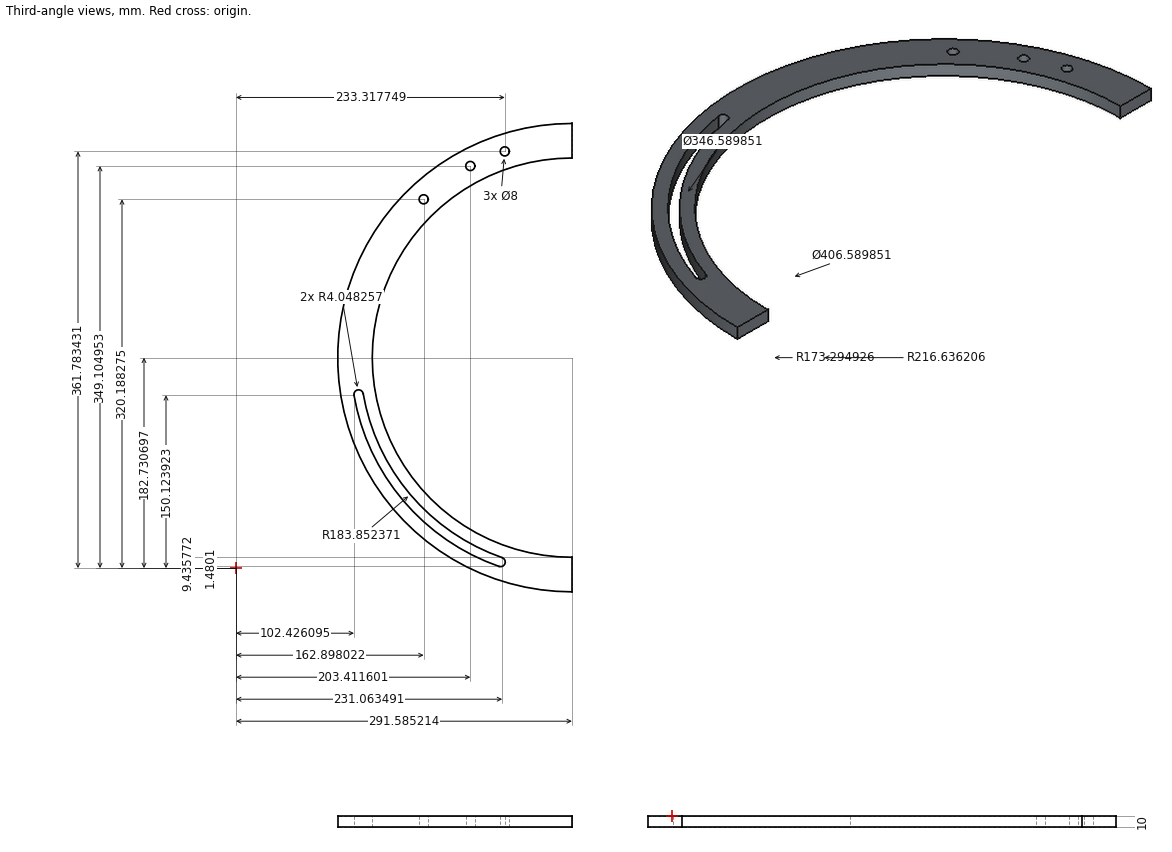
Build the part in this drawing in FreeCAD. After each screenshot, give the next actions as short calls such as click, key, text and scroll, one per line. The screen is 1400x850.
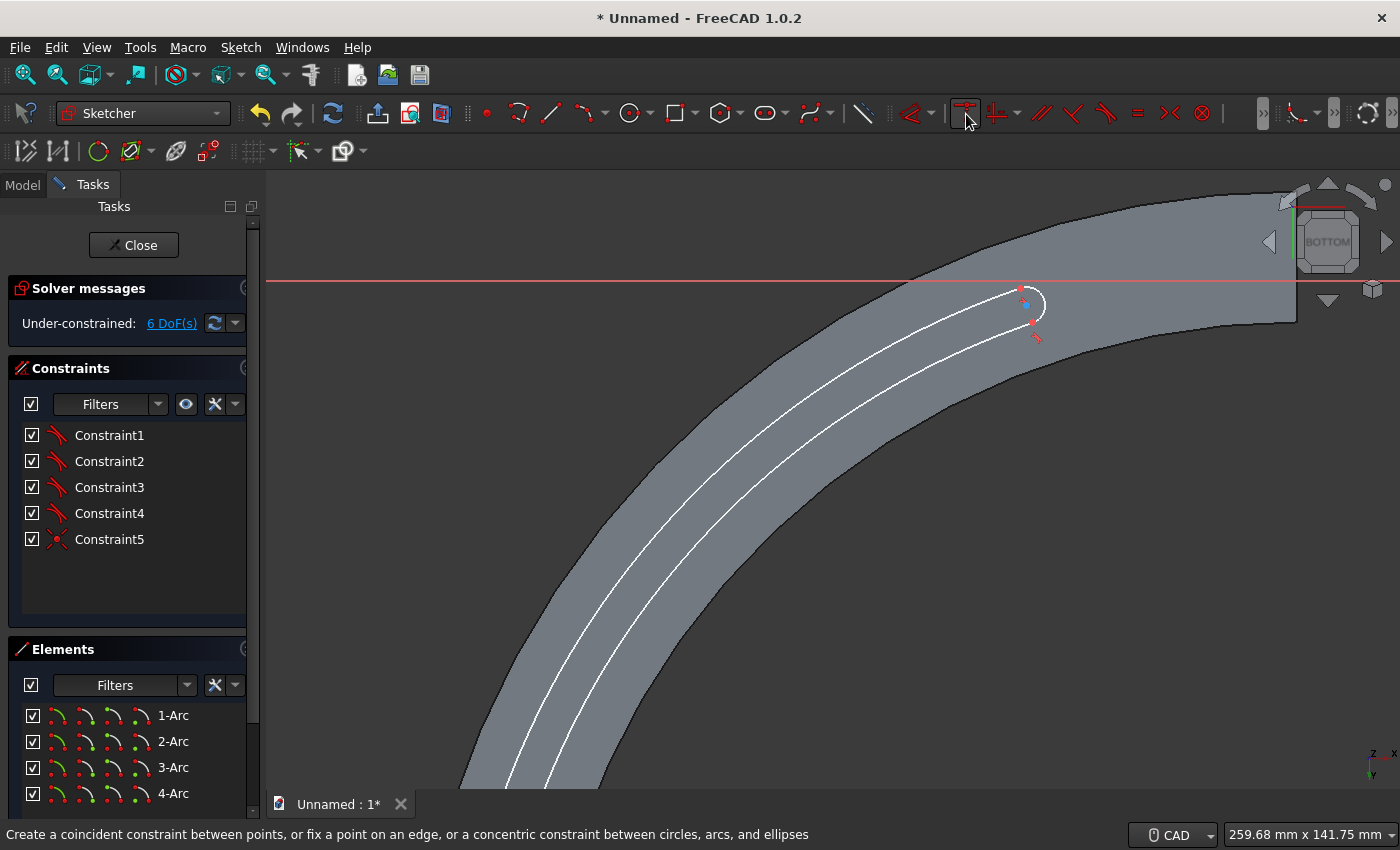
click(910, 114)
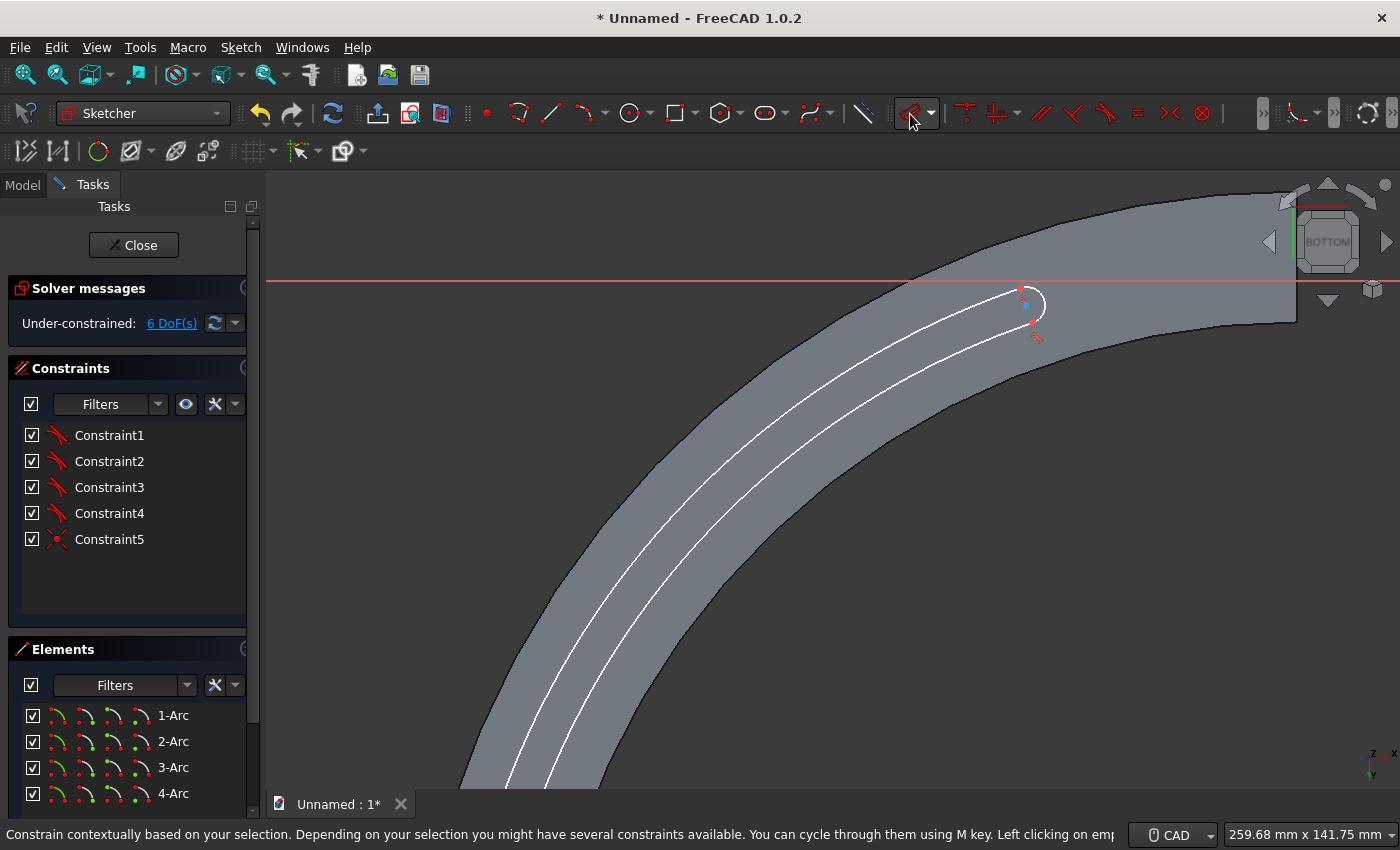
scroll(1046, 310, down, 3)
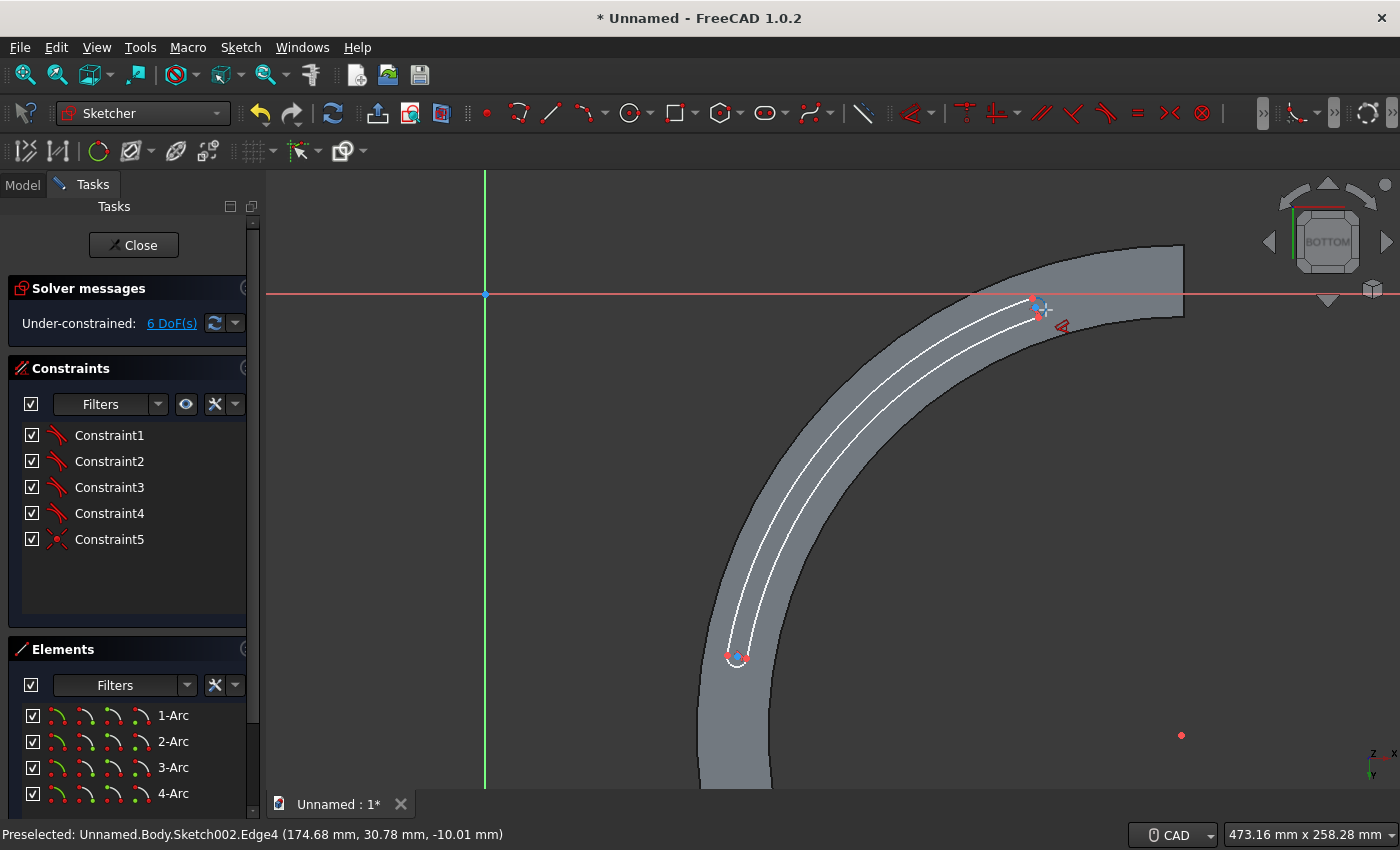
scroll(730, 664, up, 8)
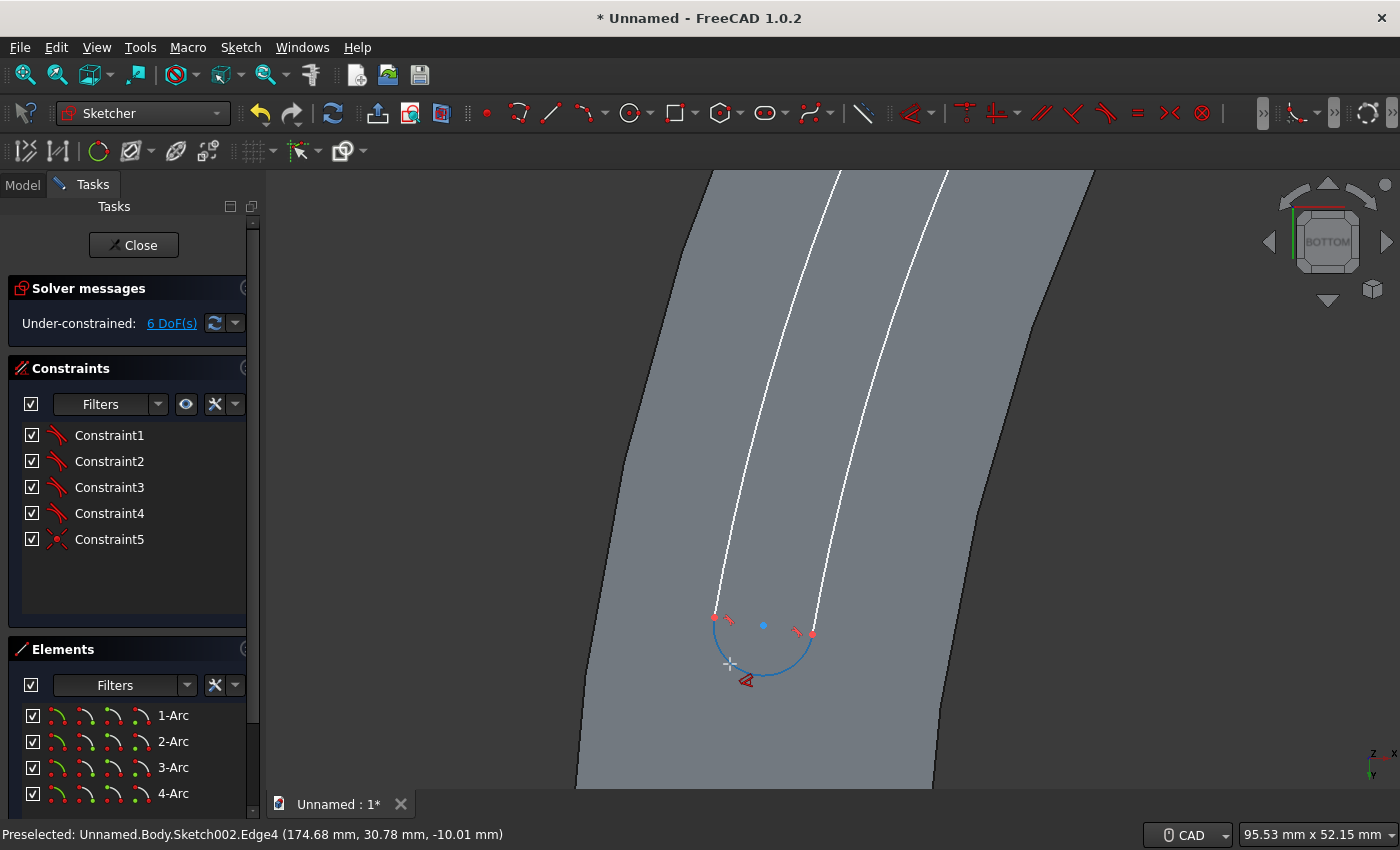
click(728, 660)
click(705, 682)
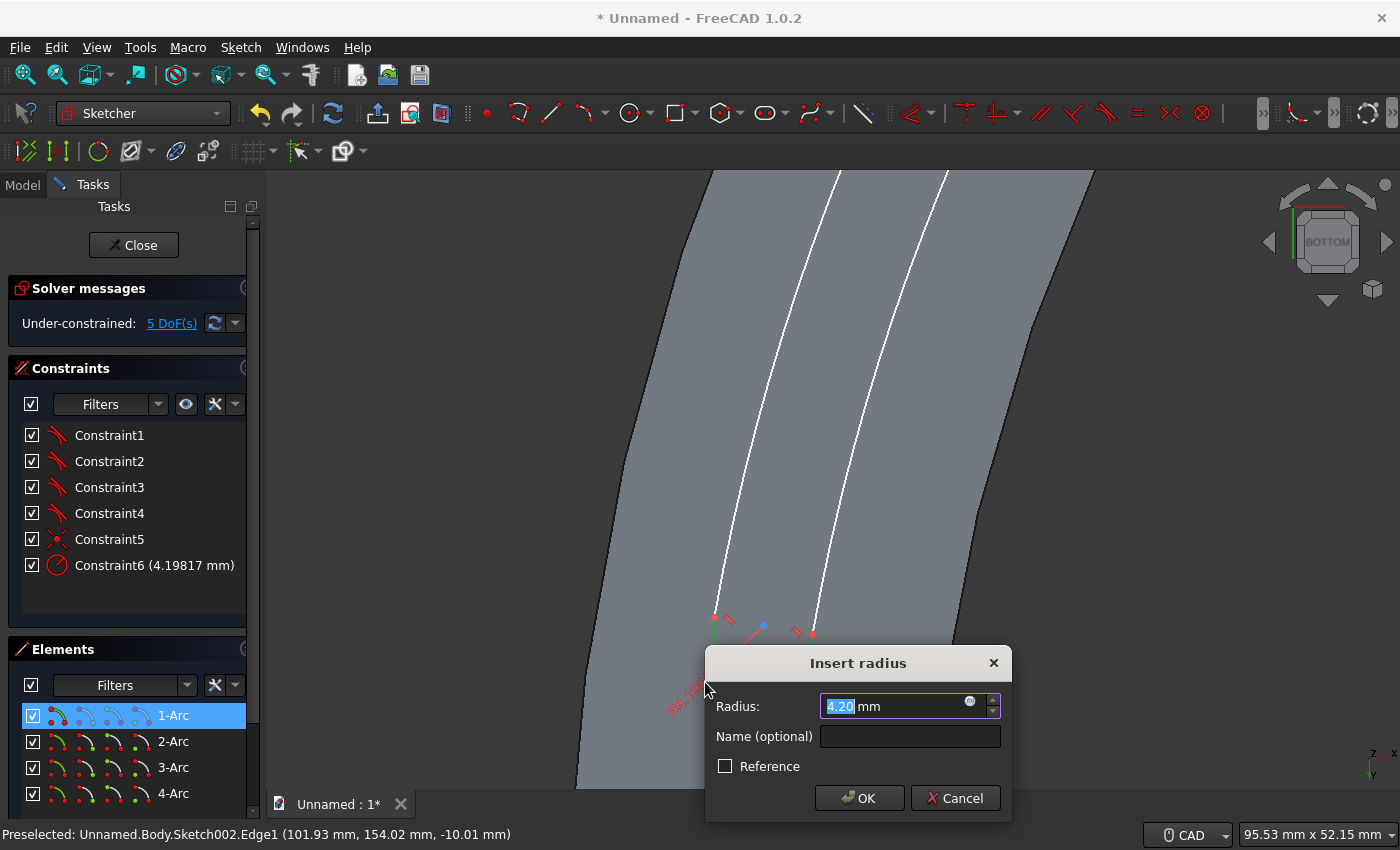
text(4.048257)
key(Return)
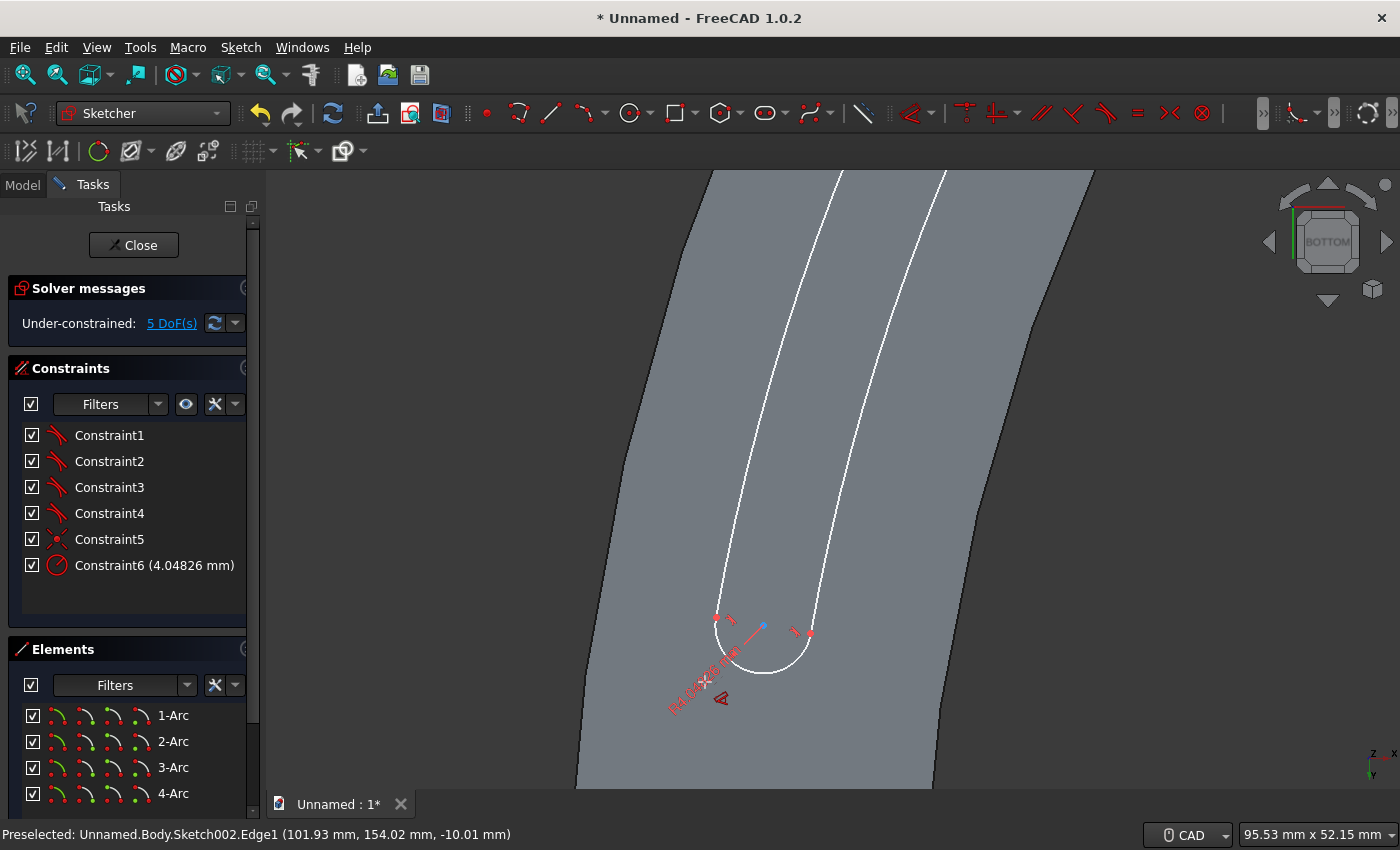
scroll(730, 664, down, 8)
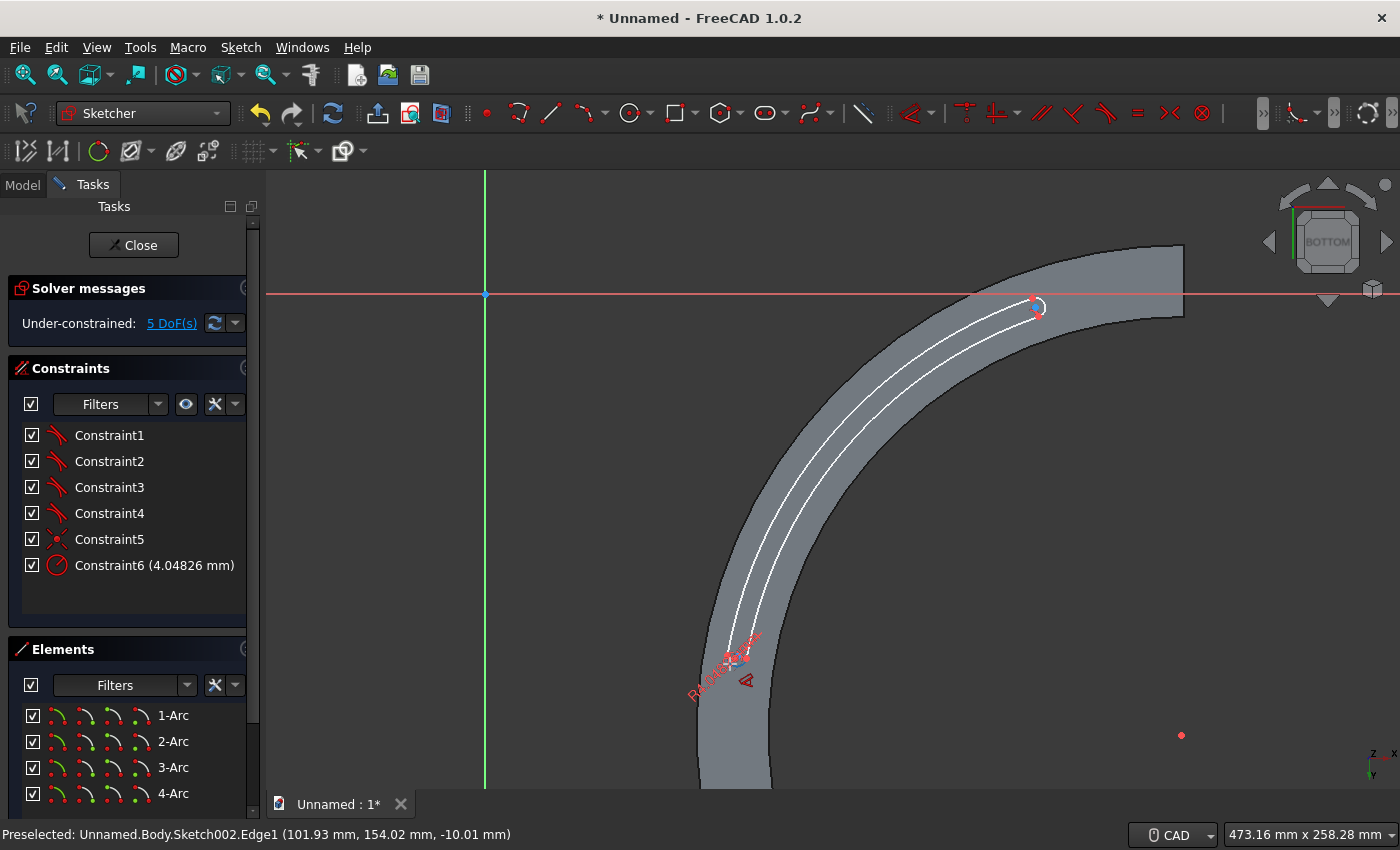
click(914, 383)
click(1111, 266)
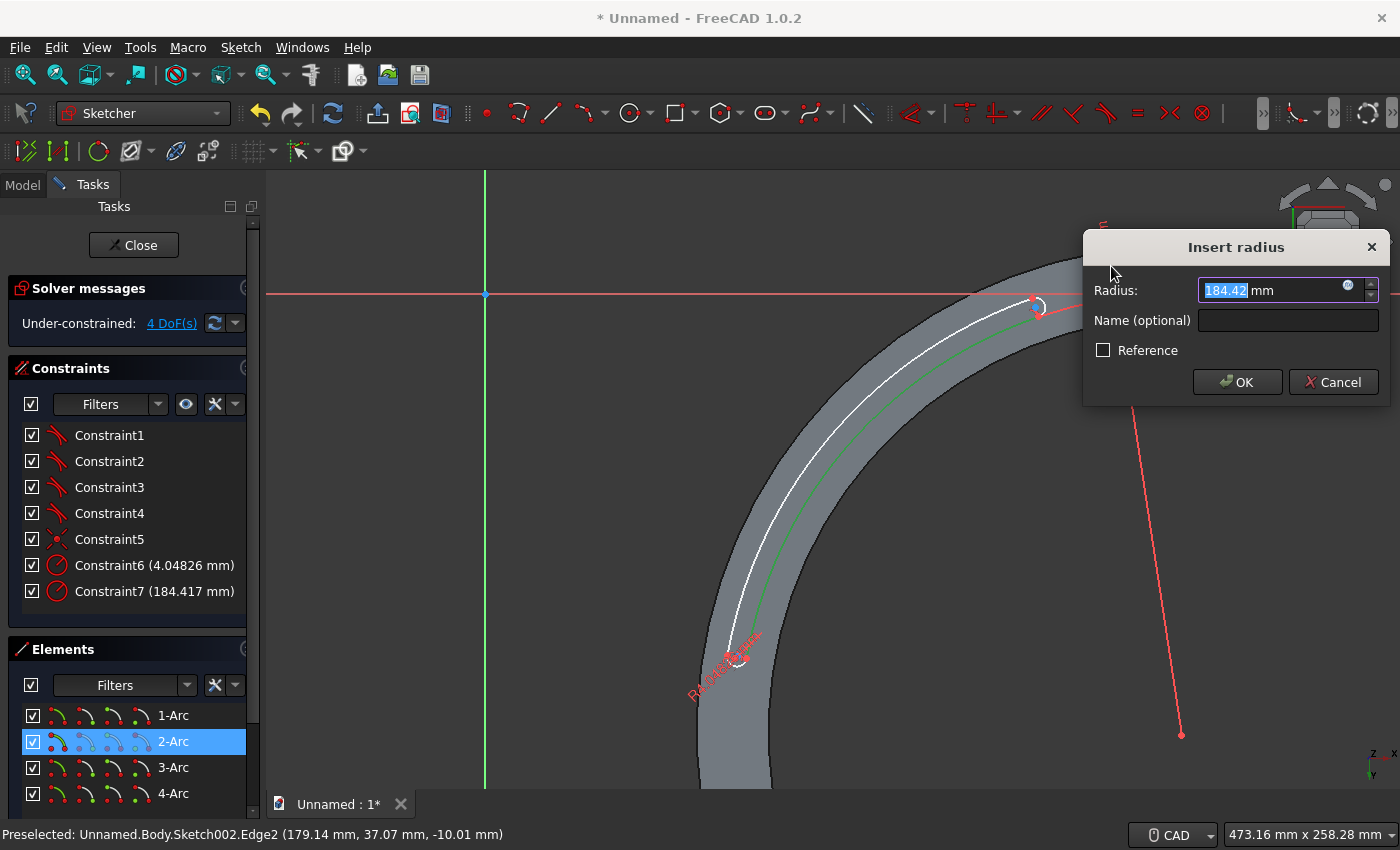
text(183.852371)
key(Return)